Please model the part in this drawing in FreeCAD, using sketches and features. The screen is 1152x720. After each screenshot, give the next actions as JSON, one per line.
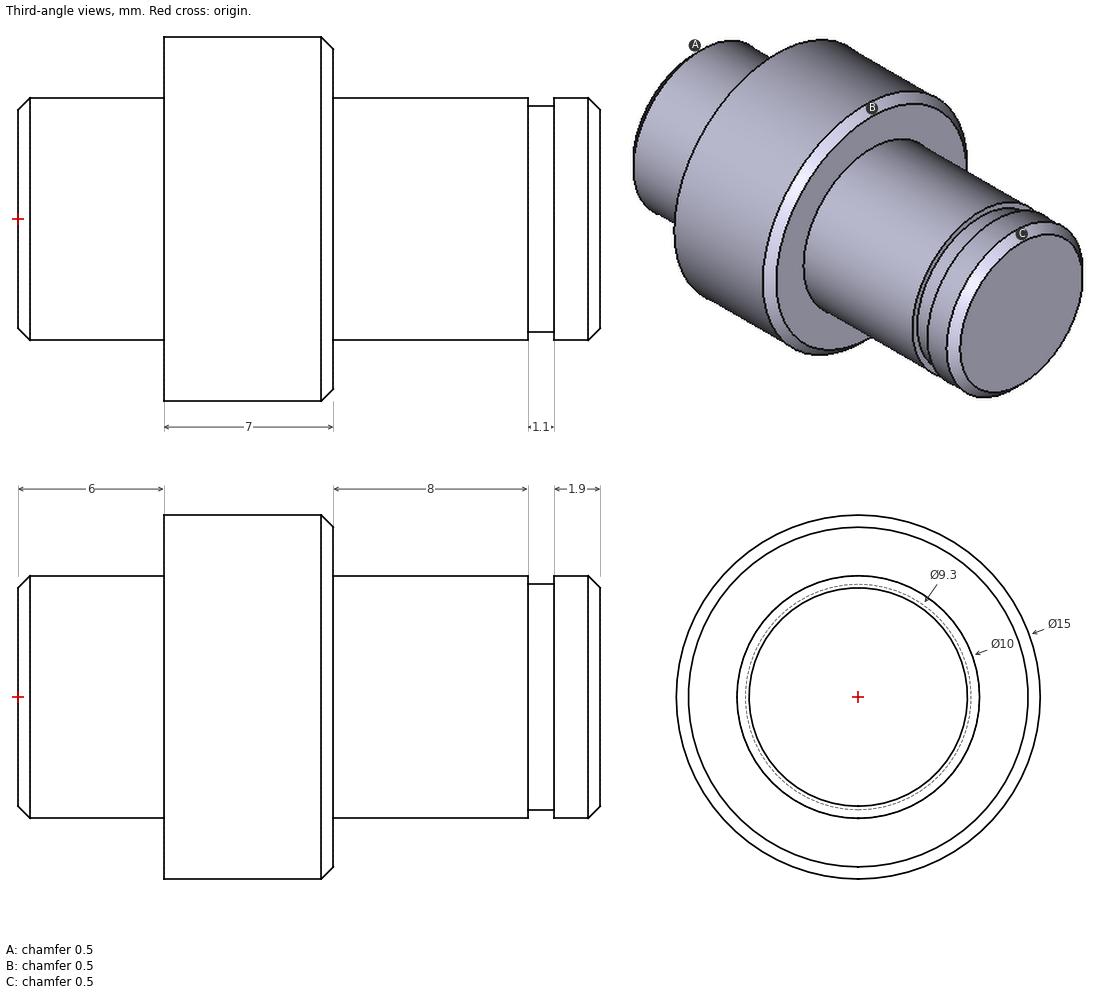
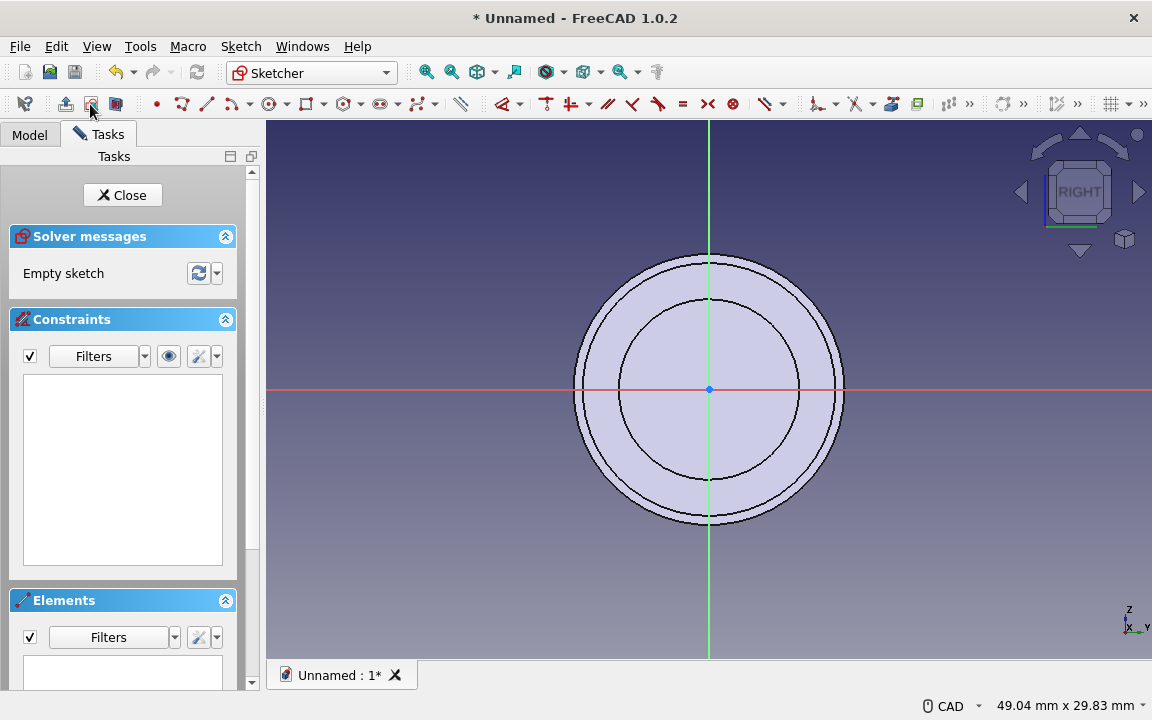
{"action": "scroll", "coordinate": [765, 389], "scroll_direction": "up", "scroll_amount": 4}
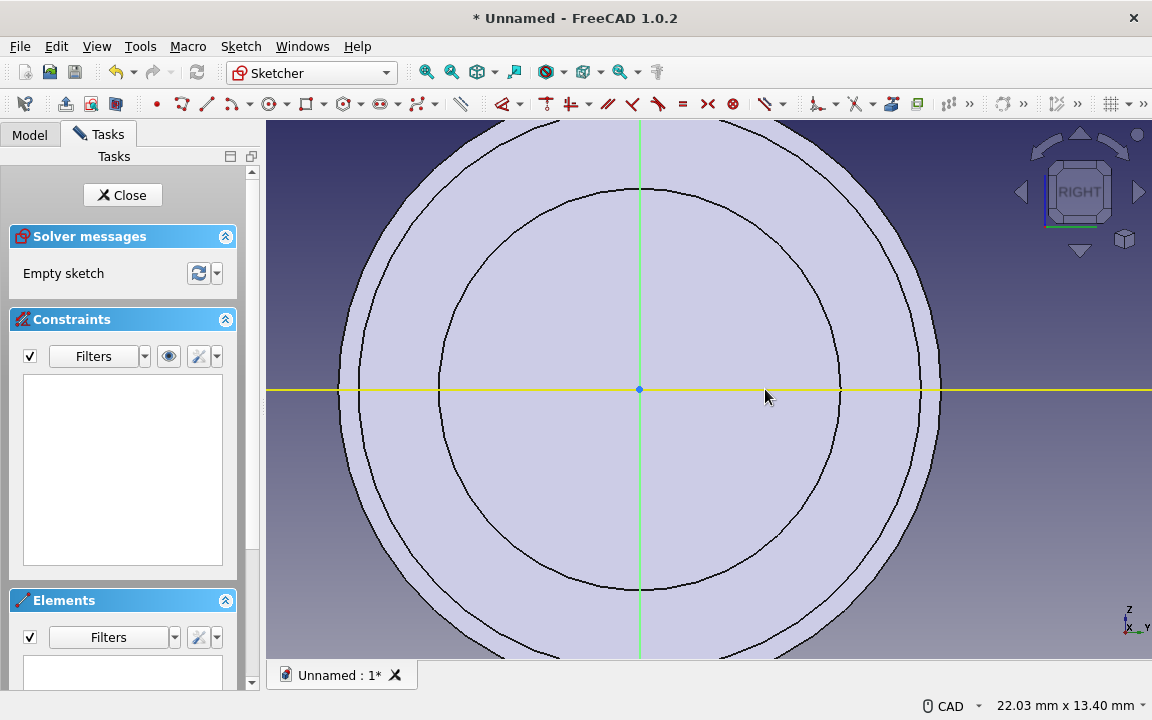
{"action": "left_click", "coordinate": [268, 104]}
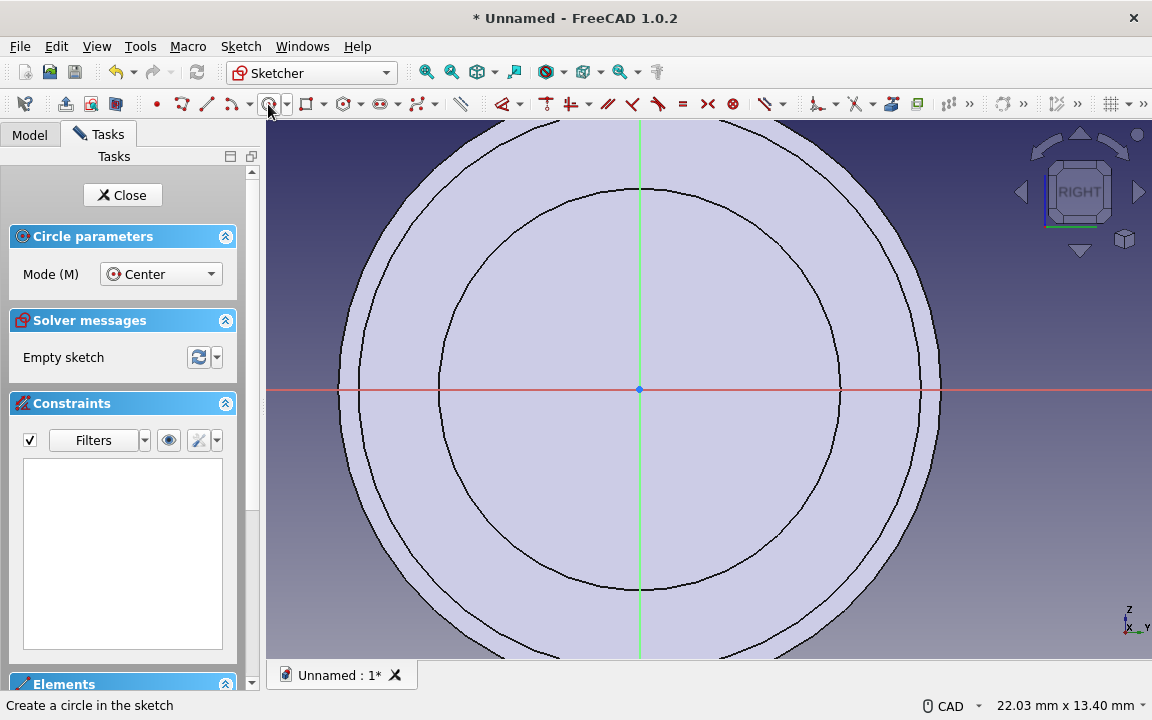
{"action": "left_click", "coordinate": [640, 389]}
{"action": "mouse_move", "coordinate": [772, 257]}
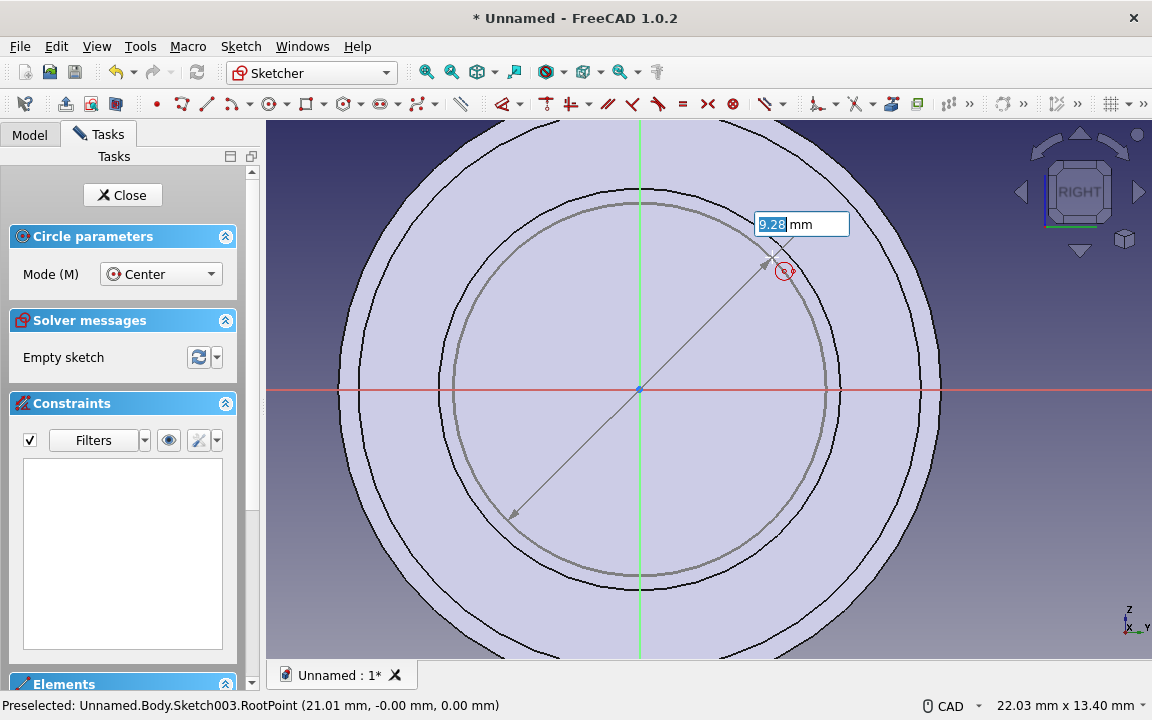
{"action": "type", "text": "9.3"}
{"action": "key", "text": "Return"}
{"action": "key", "text": "Escape"}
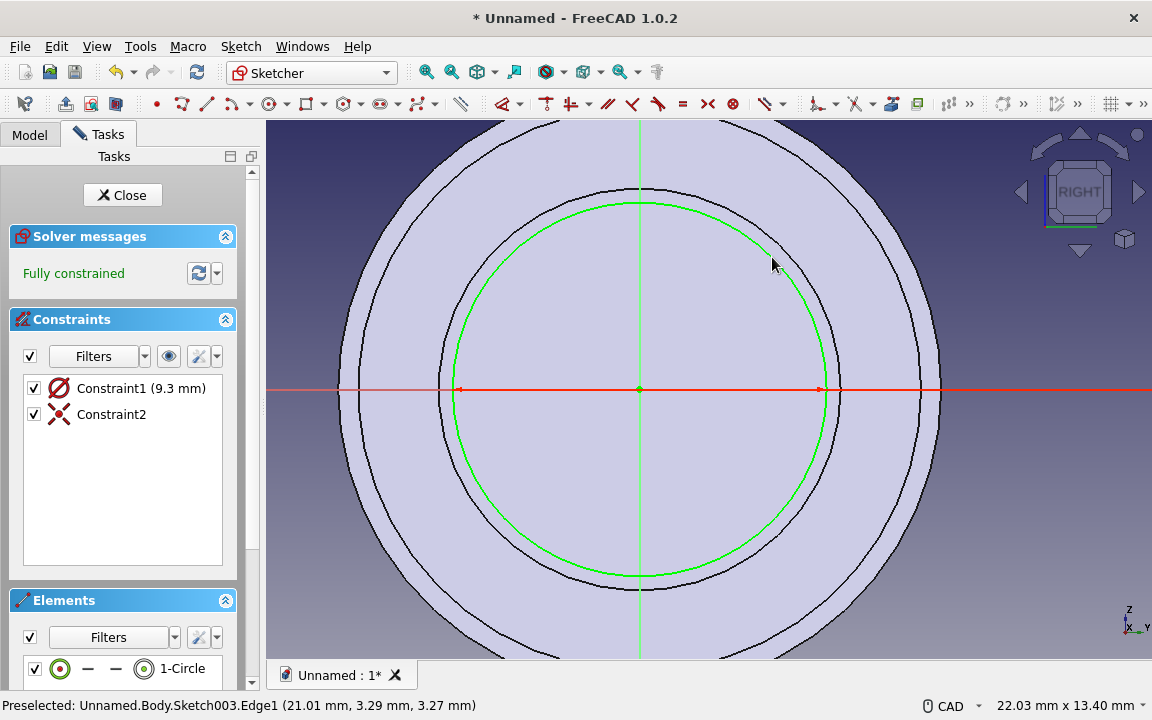
{"action": "left_click", "coordinate": [123, 195]}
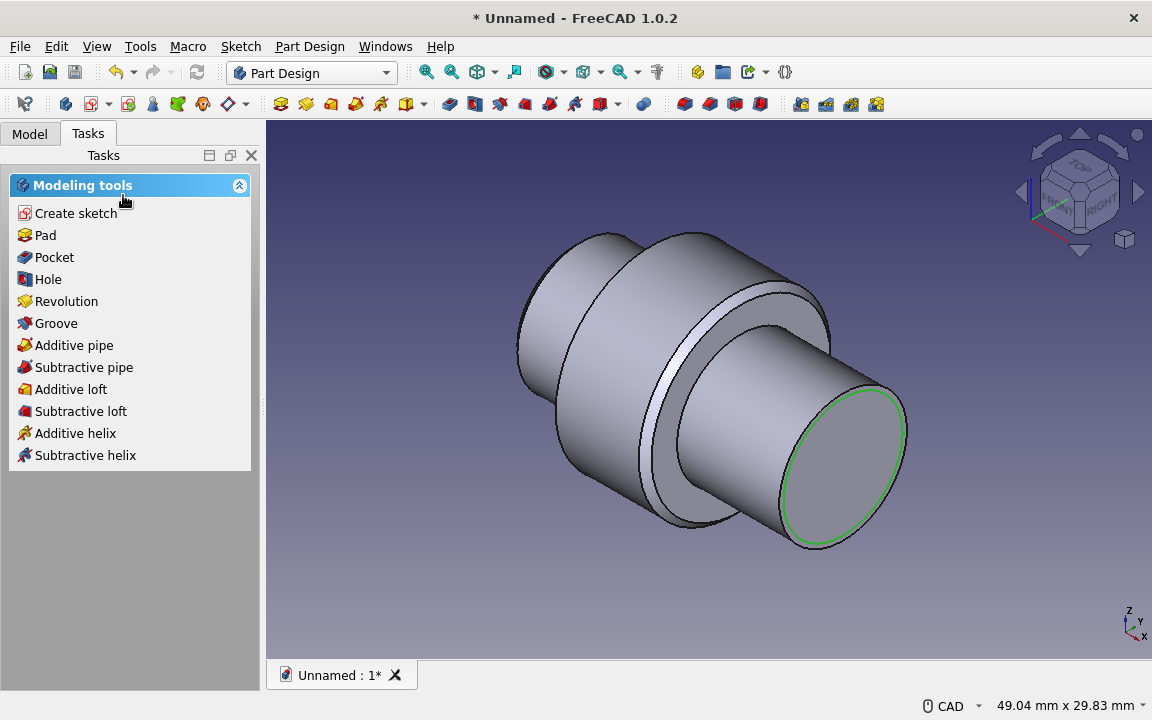
{"action": "left_click", "coordinate": [281, 104]}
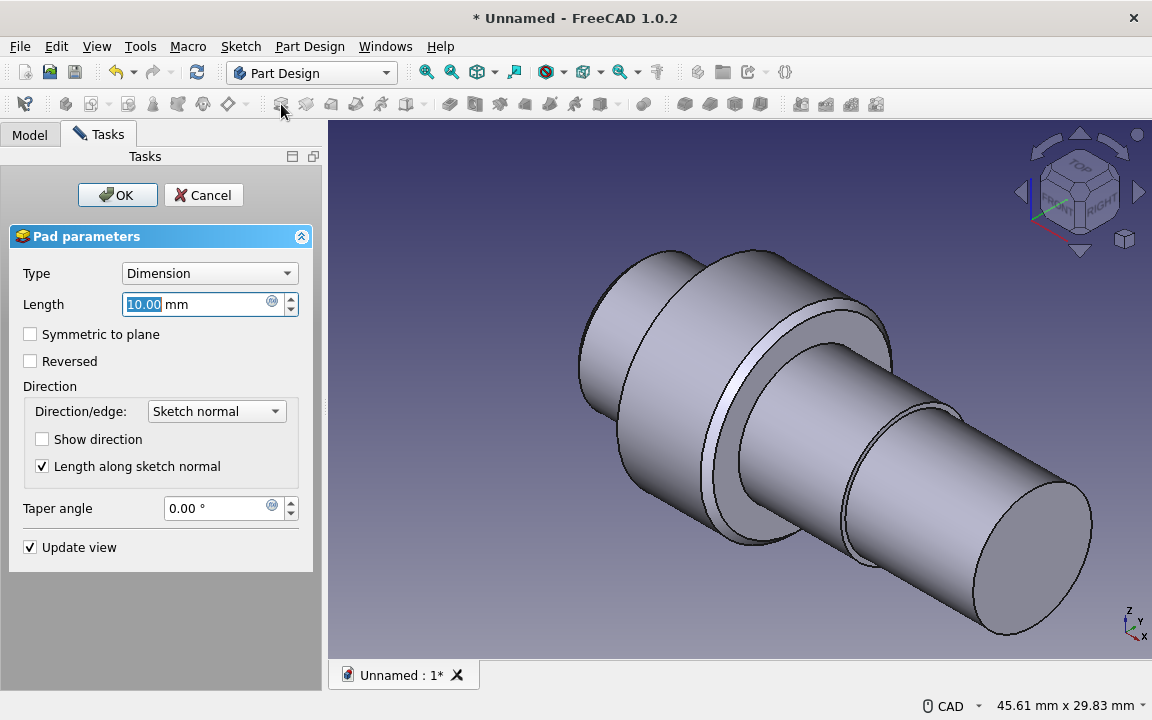
{"action": "type", "text": "1.1"}
{"action": "key", "text": "Tab"}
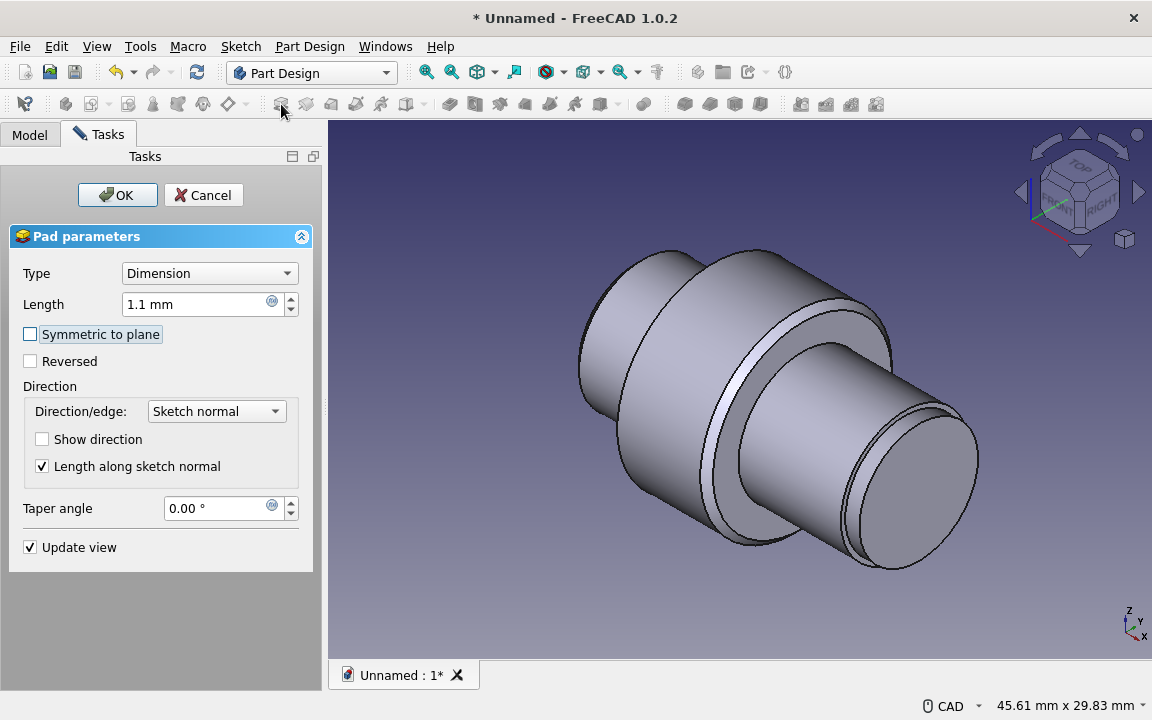
{"action": "left_click", "coordinate": [118, 195]}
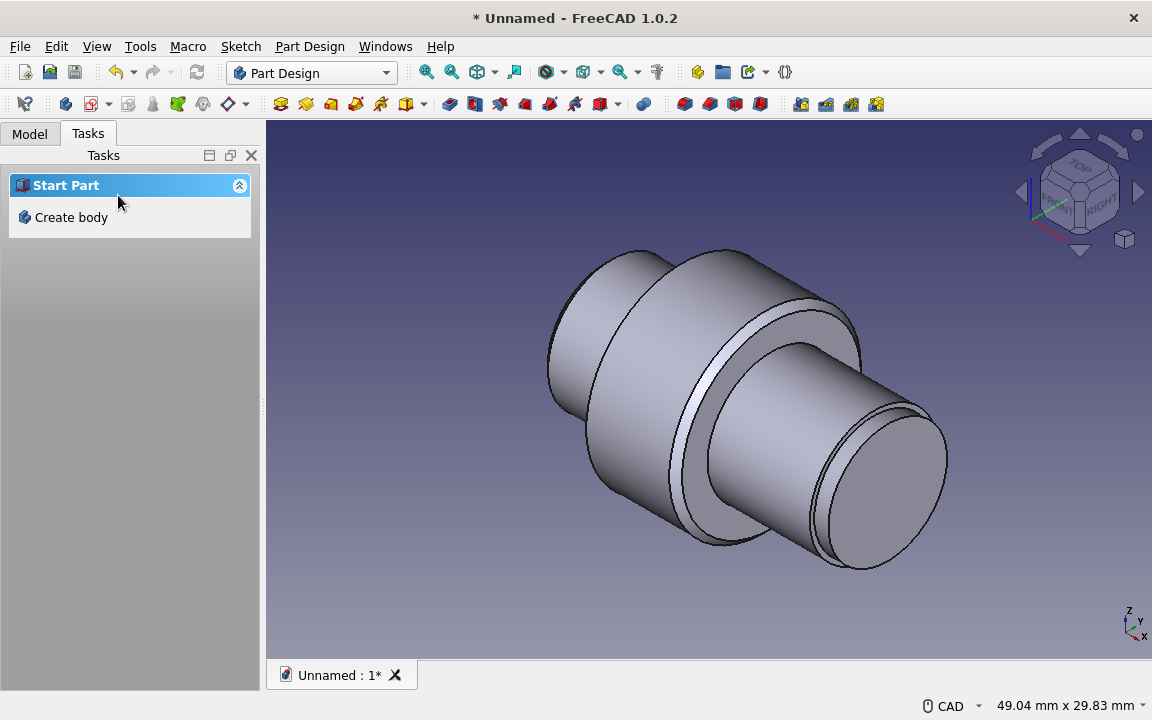
{"action": "left_click", "coordinate": [888, 492]}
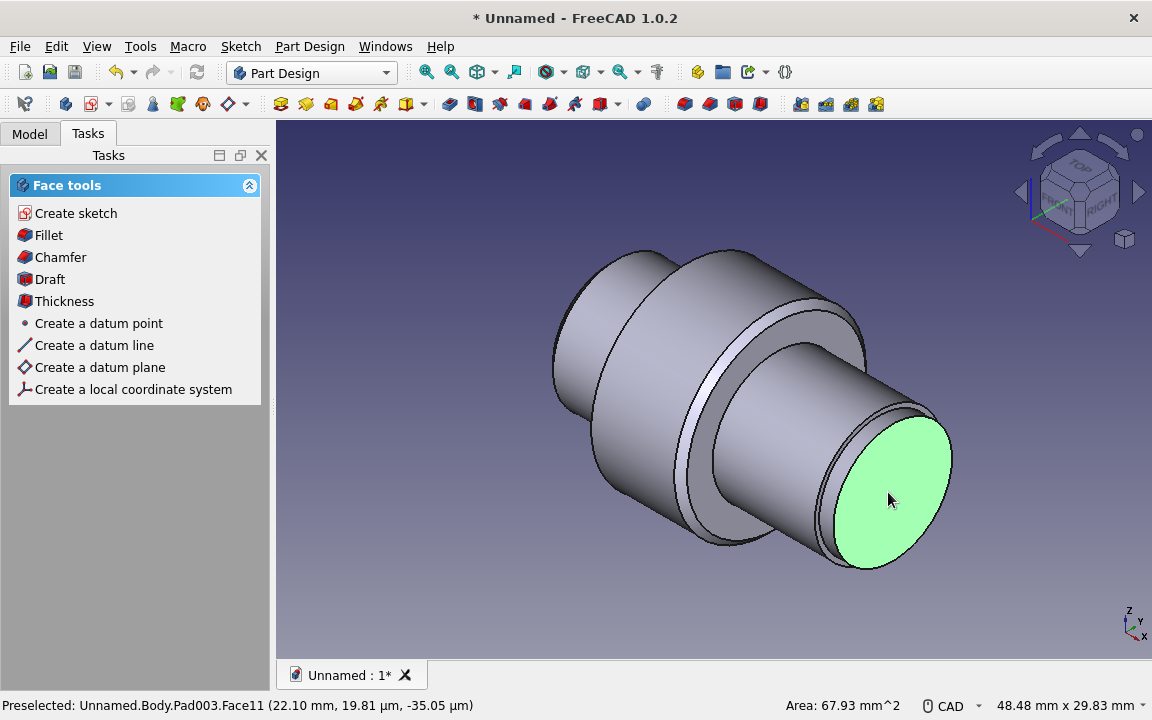
{"action": "left_click", "coordinate": [90, 104]}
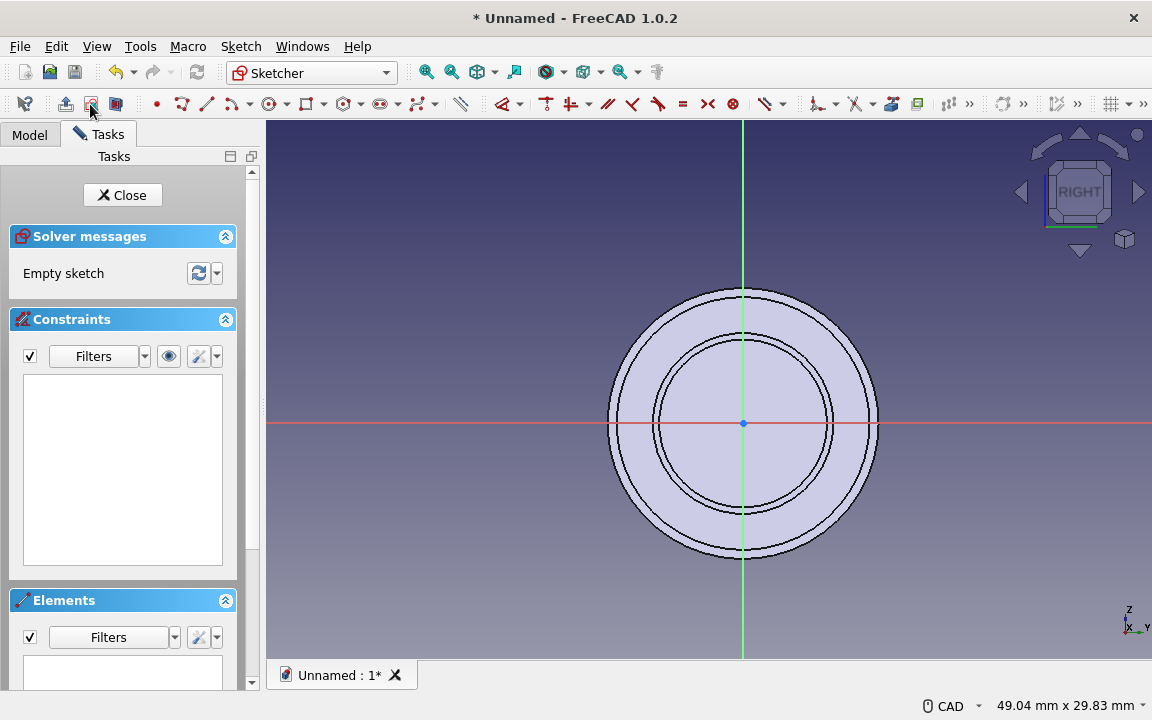
{"action": "scroll", "coordinate": [868, 465], "scroll_direction": "up", "scroll_amount": 3}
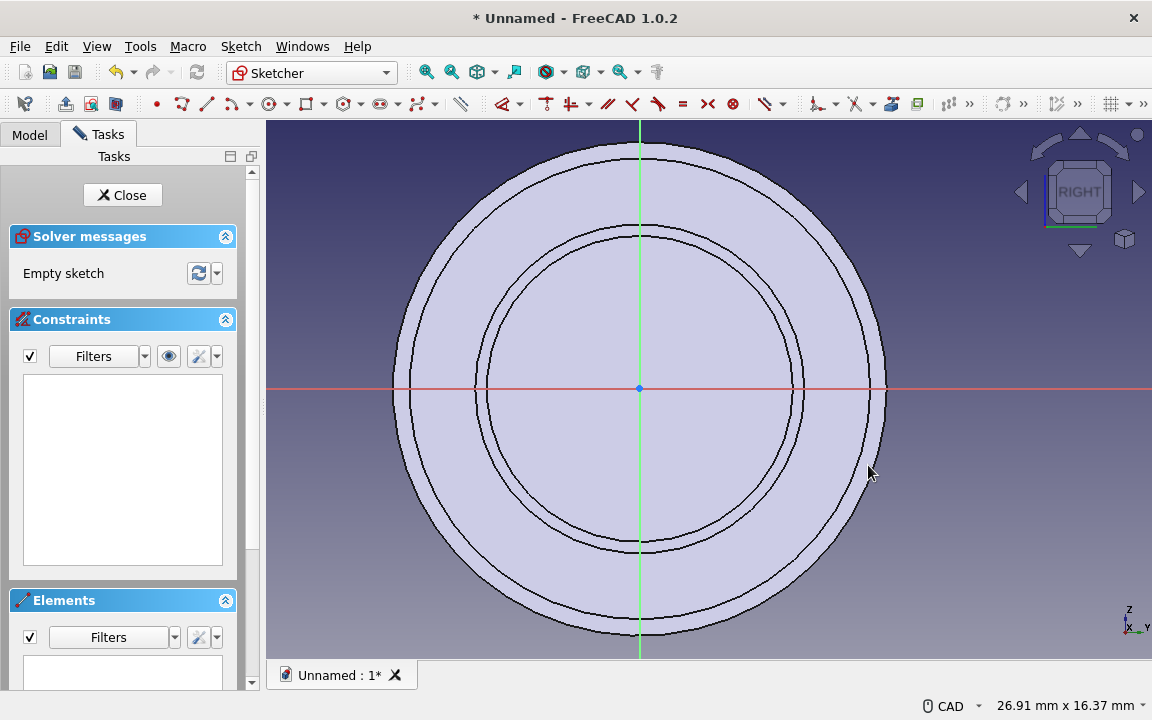
{"action": "left_click", "coordinate": [268, 104]}